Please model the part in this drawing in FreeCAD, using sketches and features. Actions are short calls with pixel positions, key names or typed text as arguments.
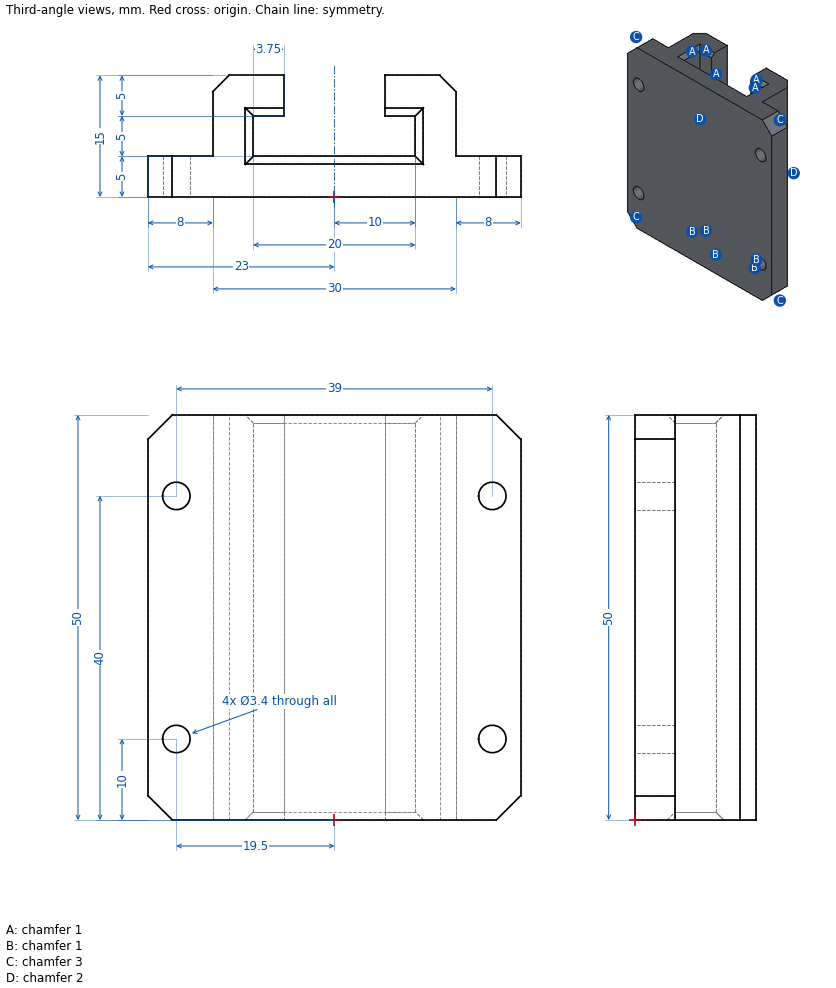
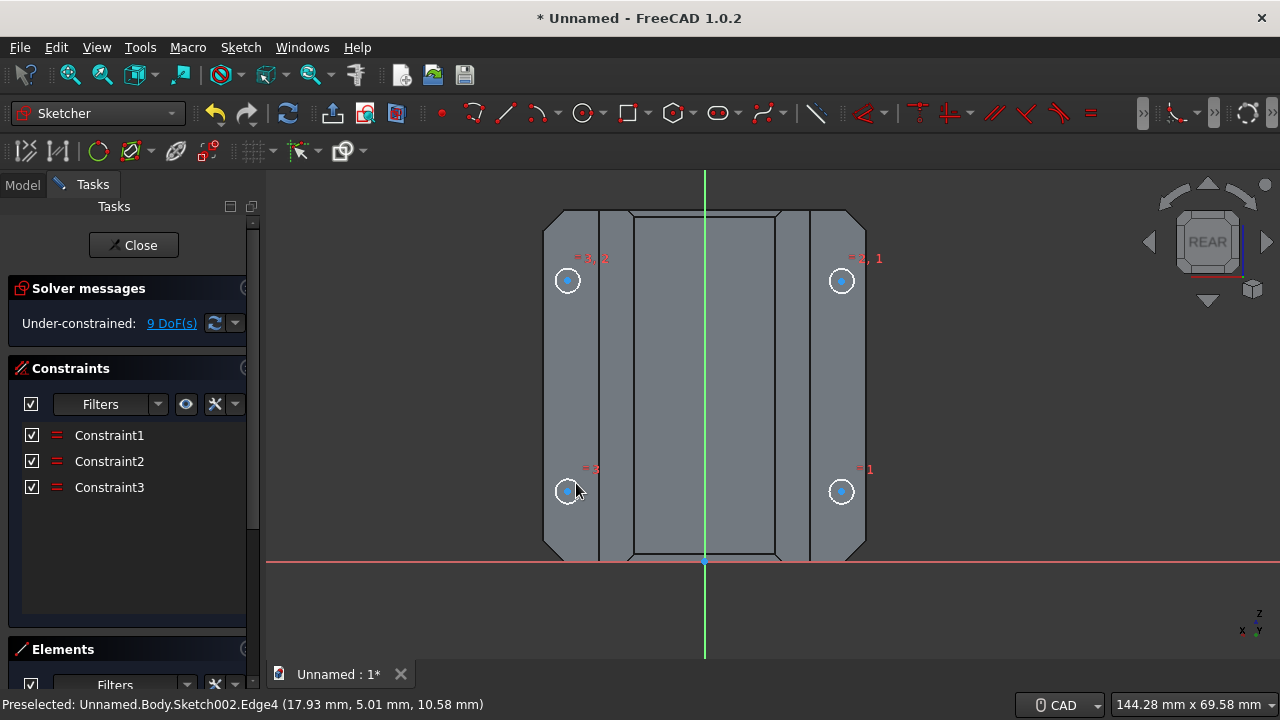
click(842, 492)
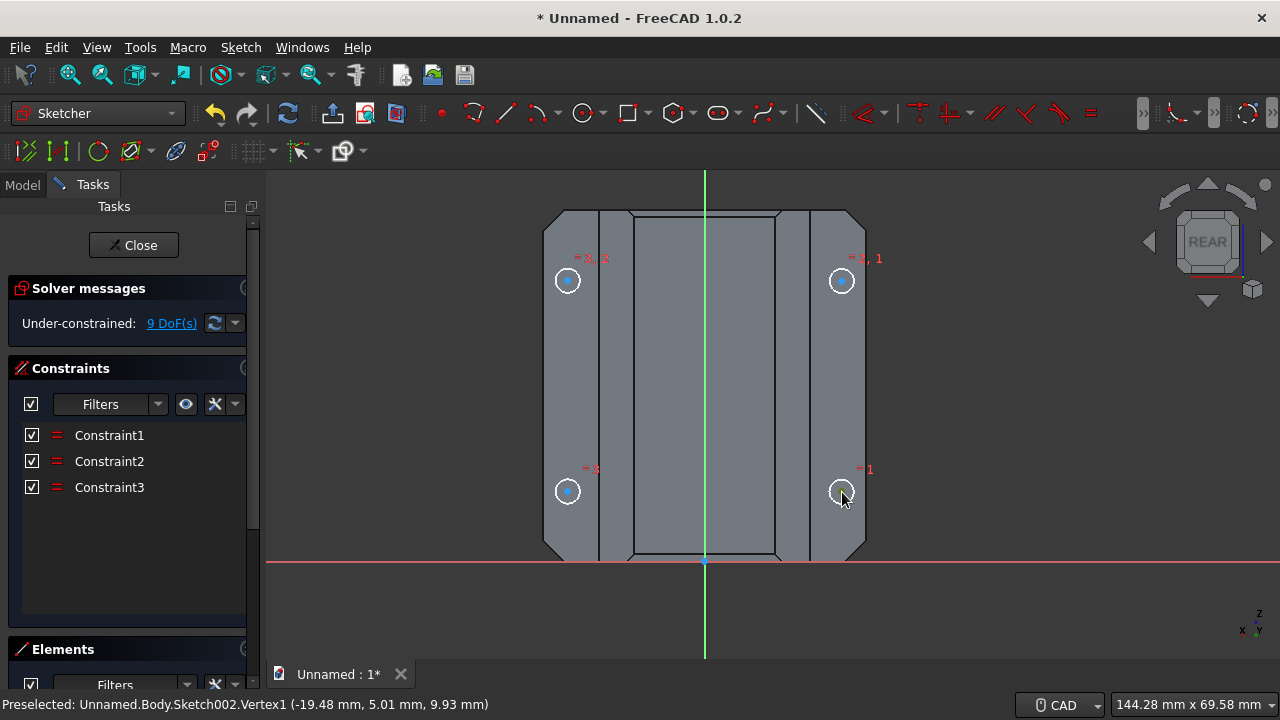
click(842, 281)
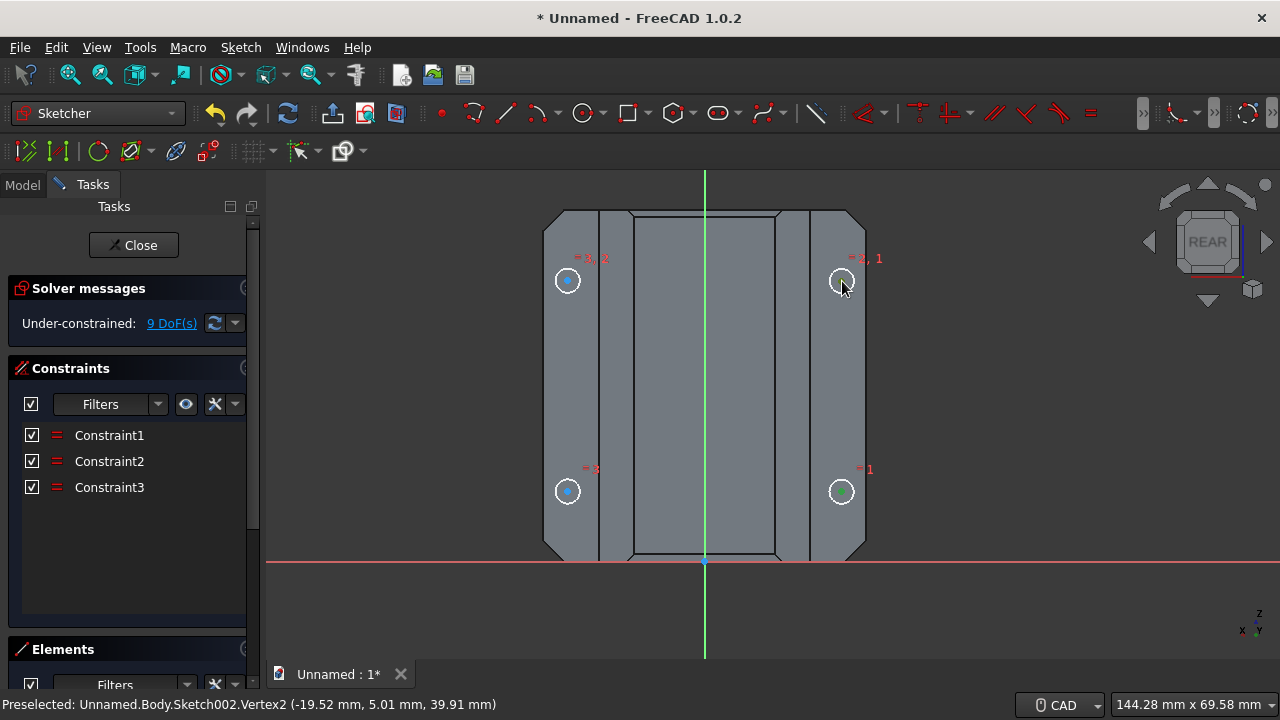
key(v)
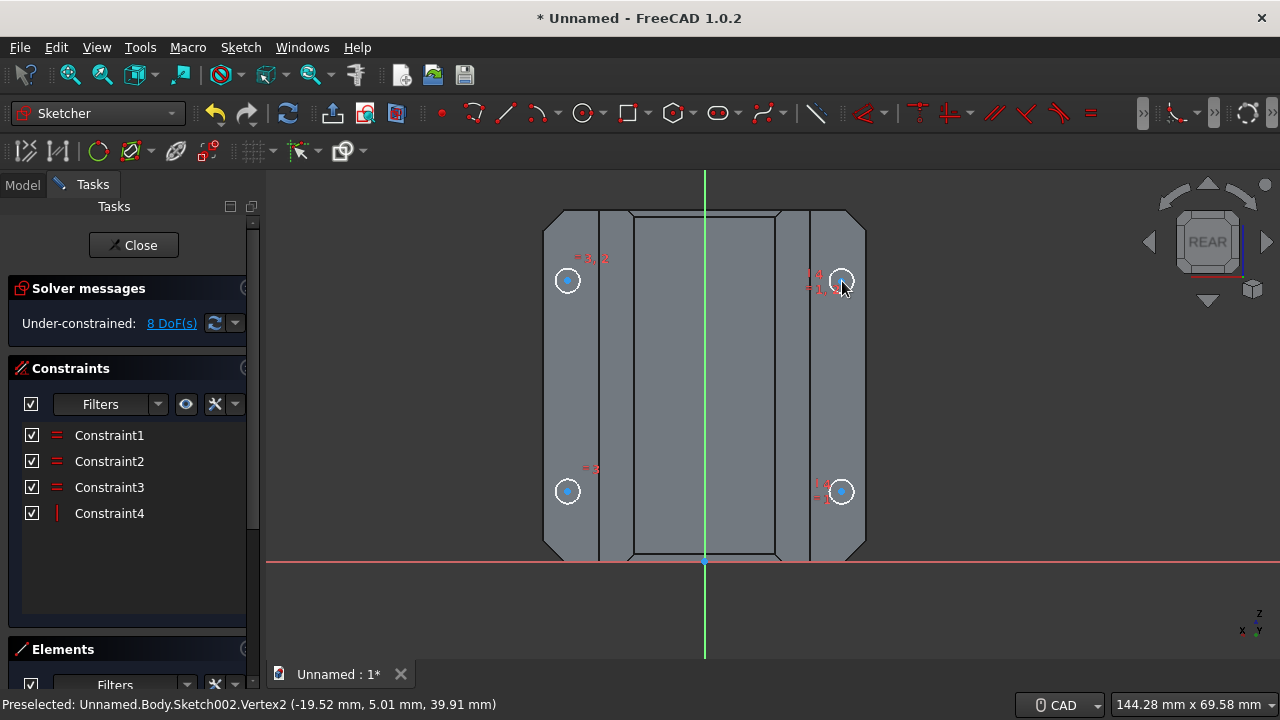
click(842, 281)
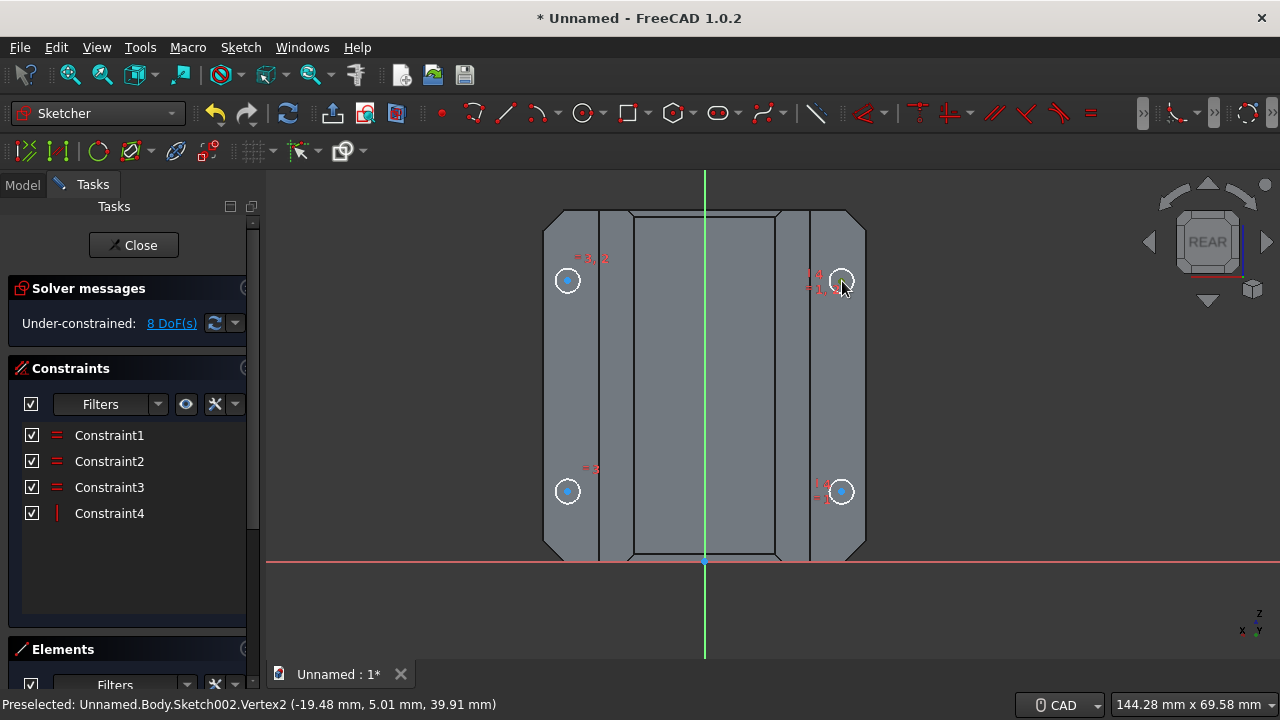
click(568, 281)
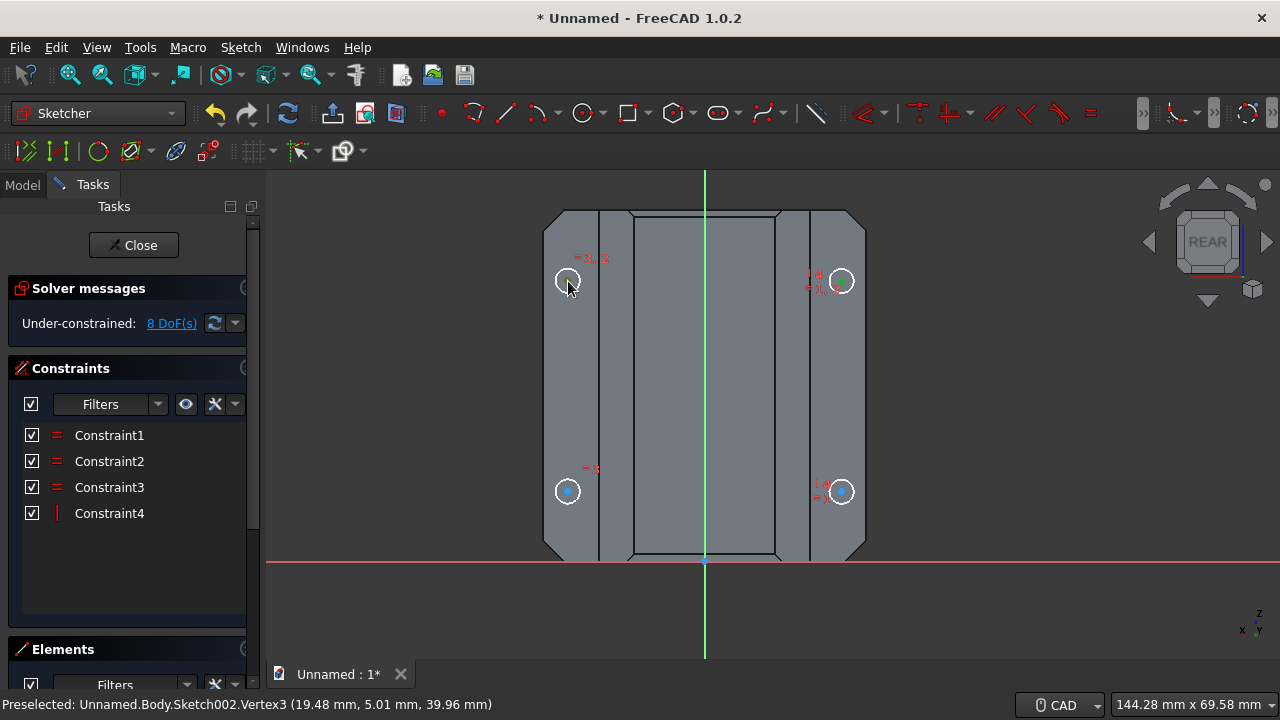
key(h)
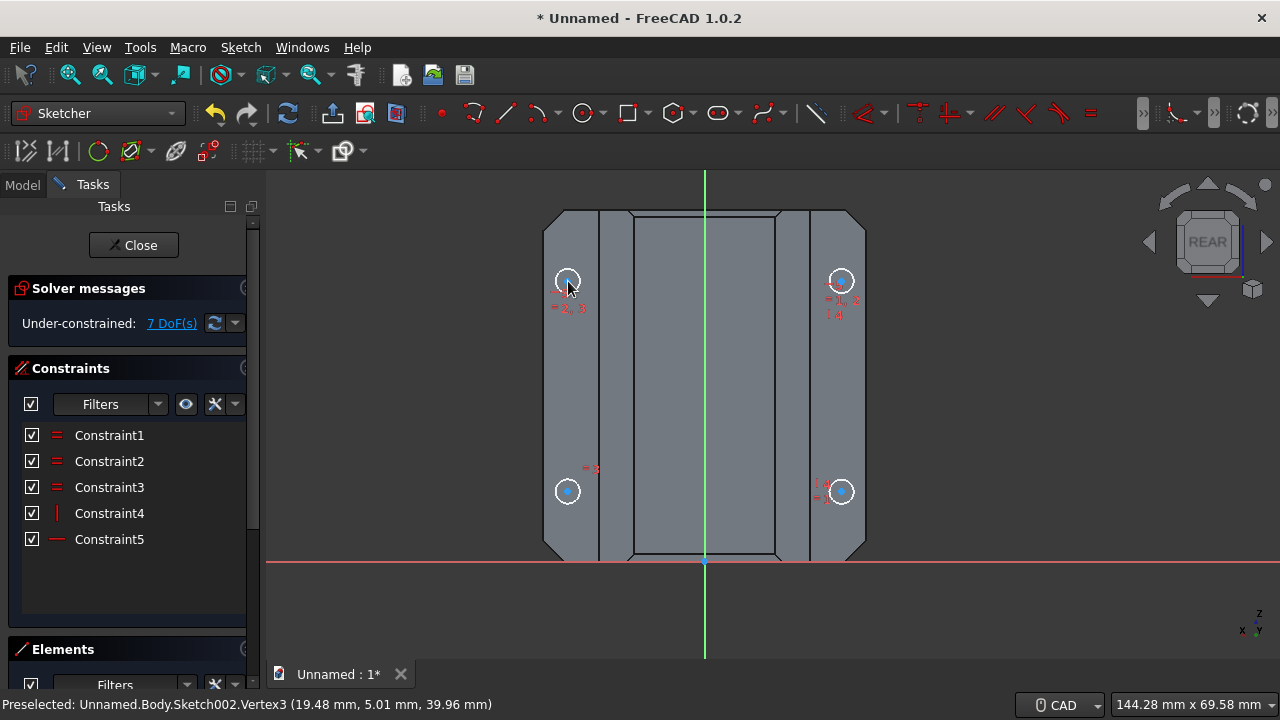
click(568, 281)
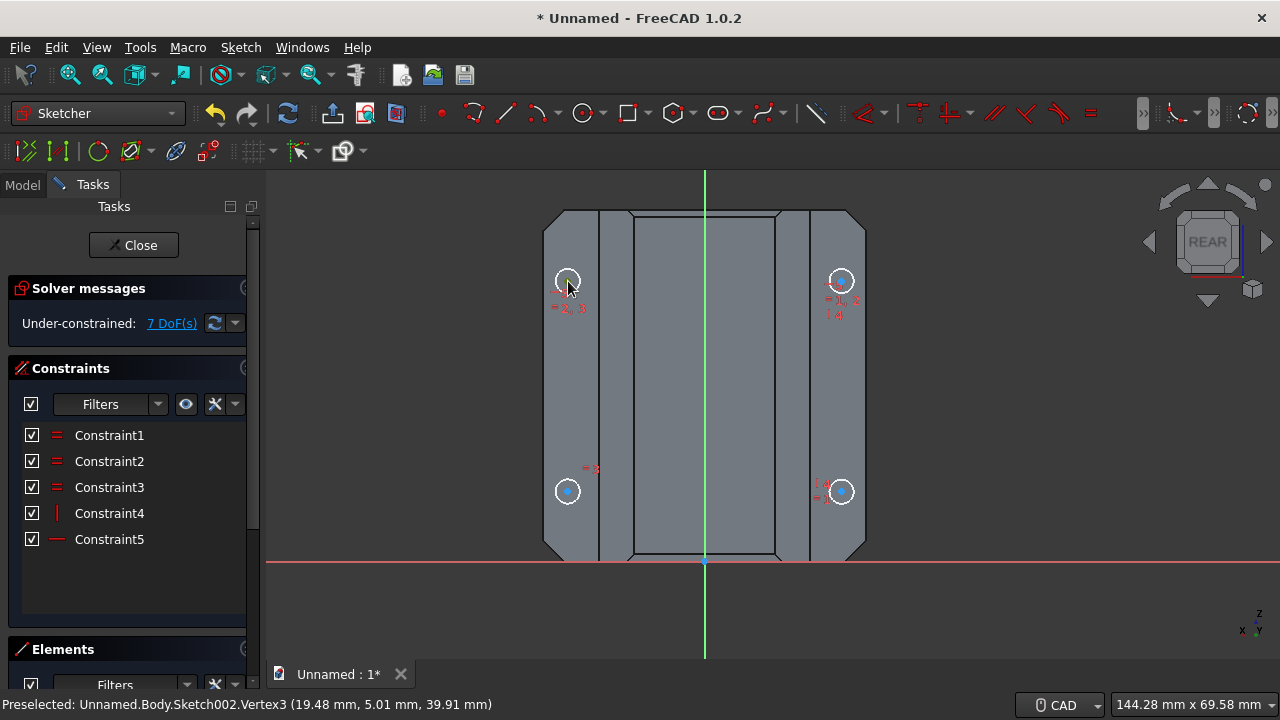
click(568, 491)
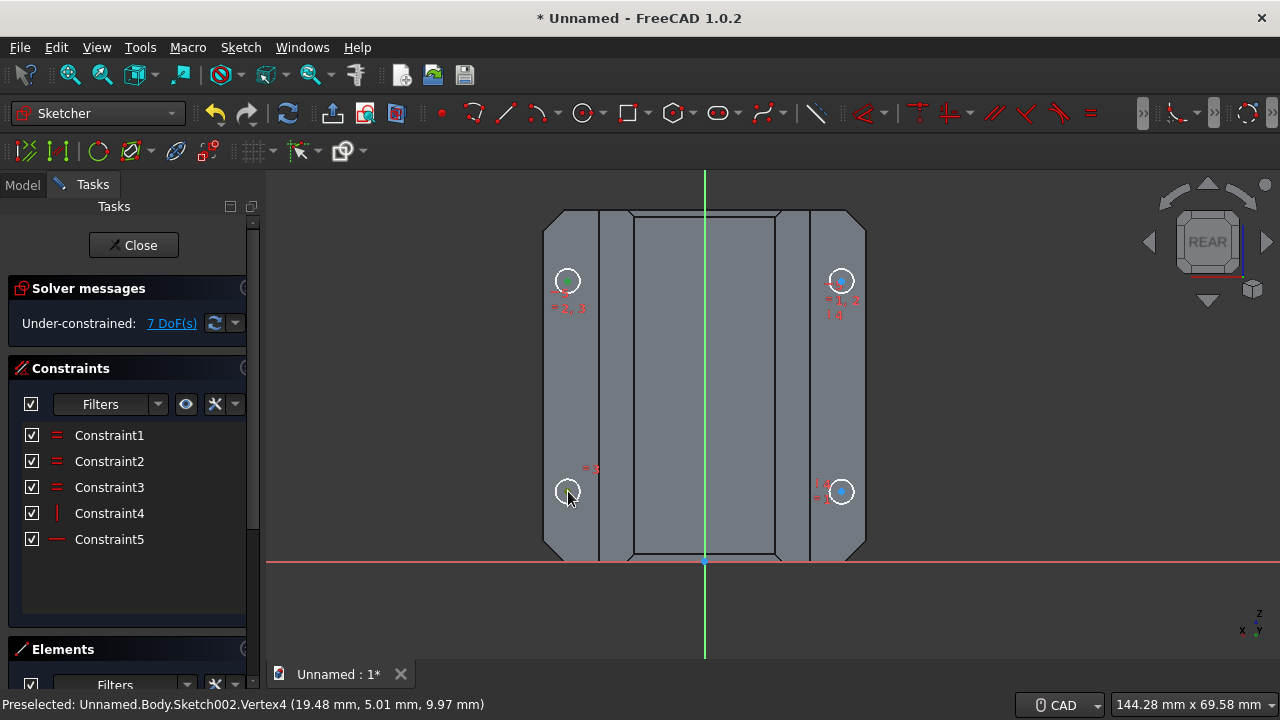
key(v)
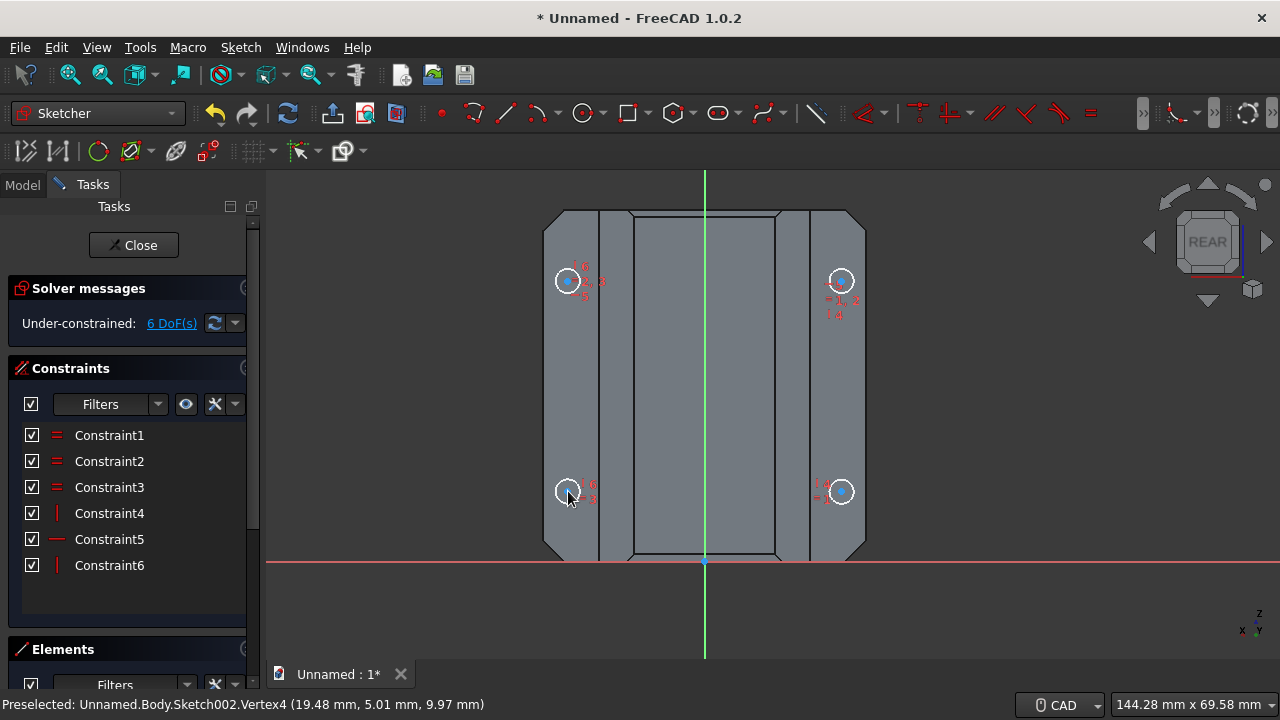
click(842, 492)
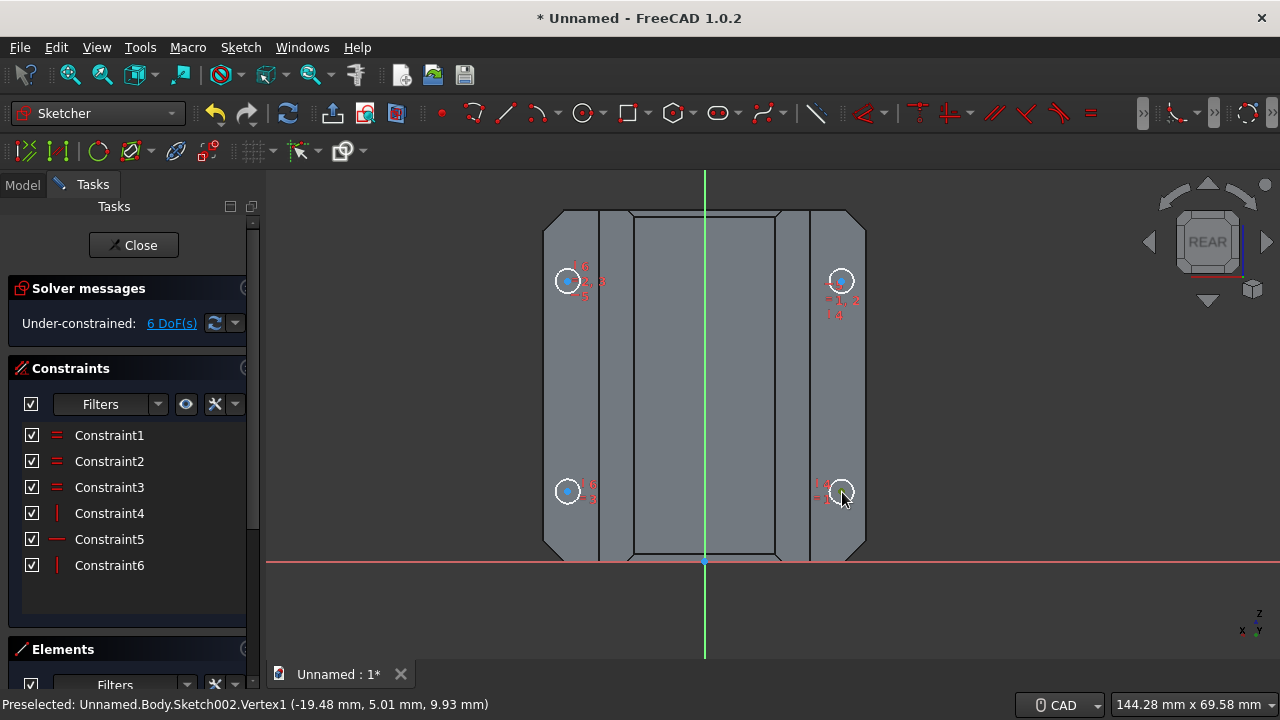
click(568, 491)